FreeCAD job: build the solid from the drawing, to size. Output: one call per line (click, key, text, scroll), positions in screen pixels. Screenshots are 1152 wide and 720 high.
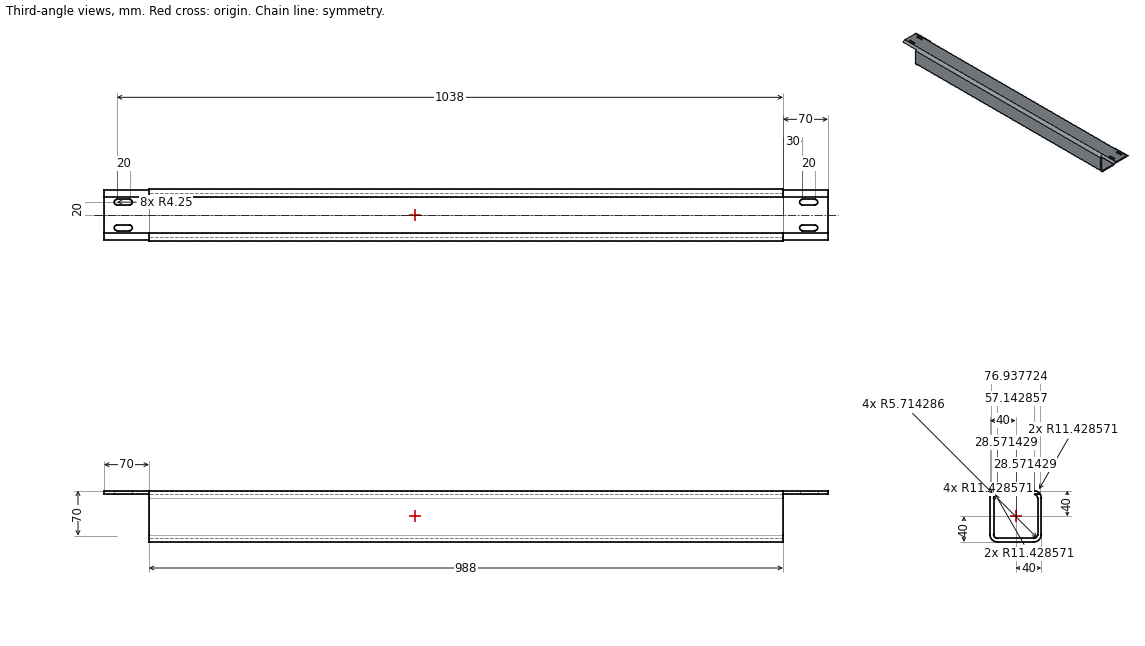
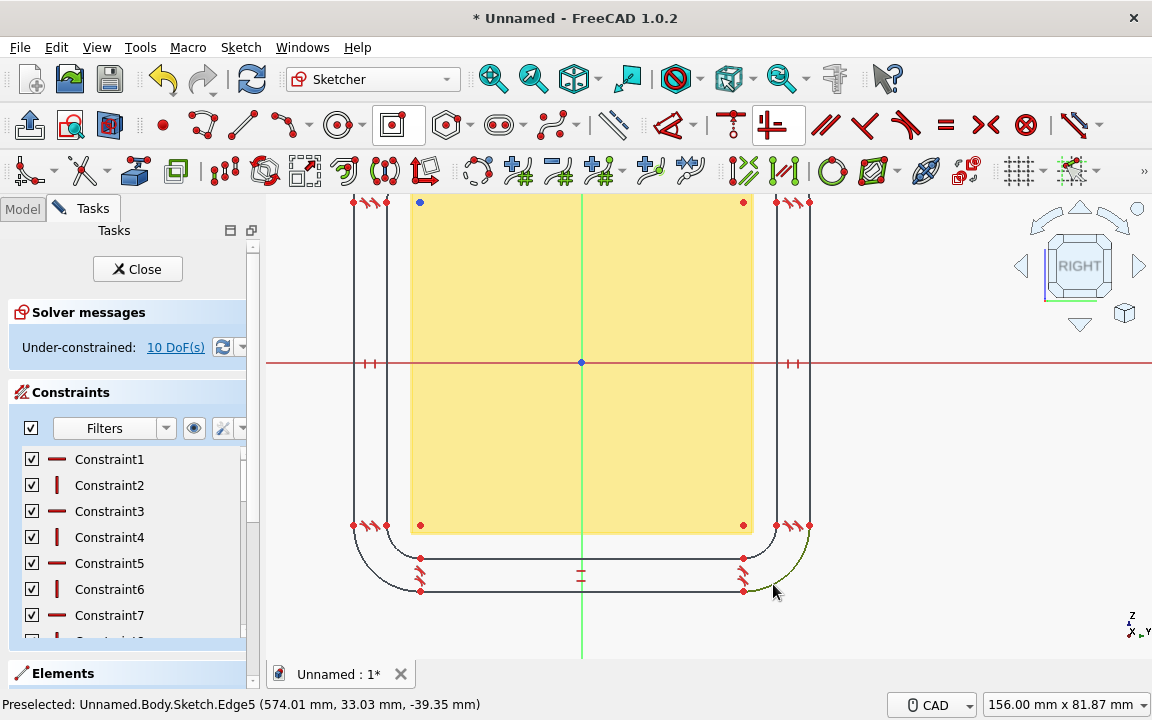
scroll(760, 556, down, 2)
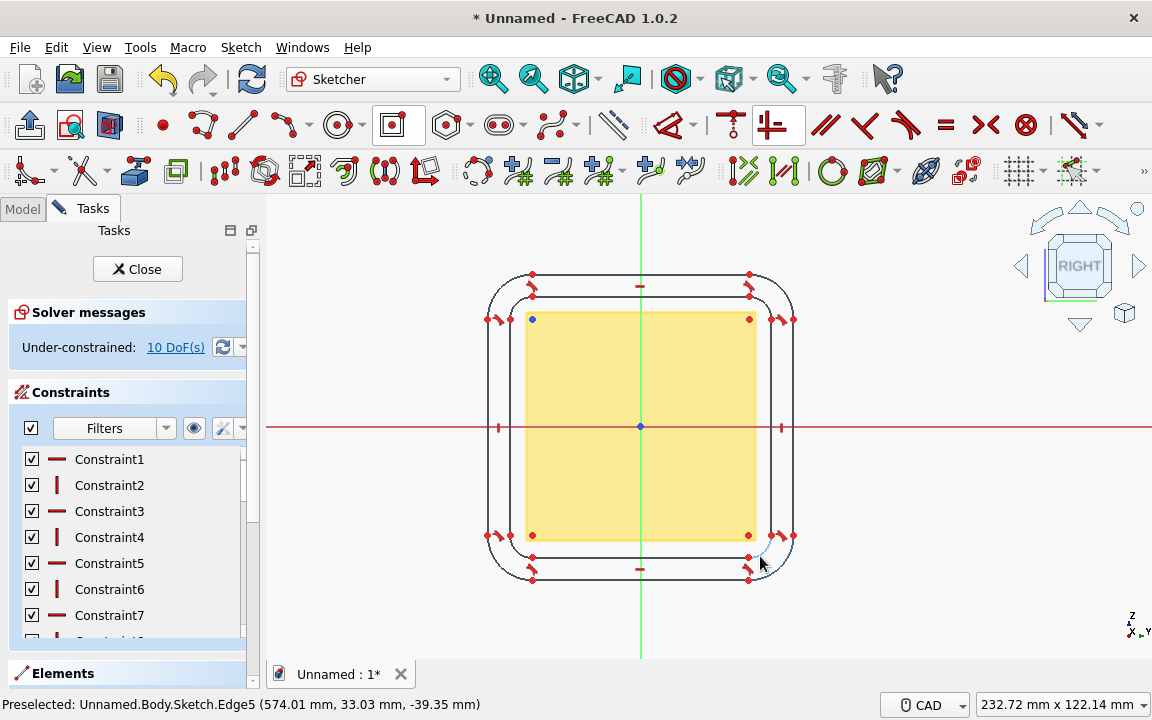
click(789, 299)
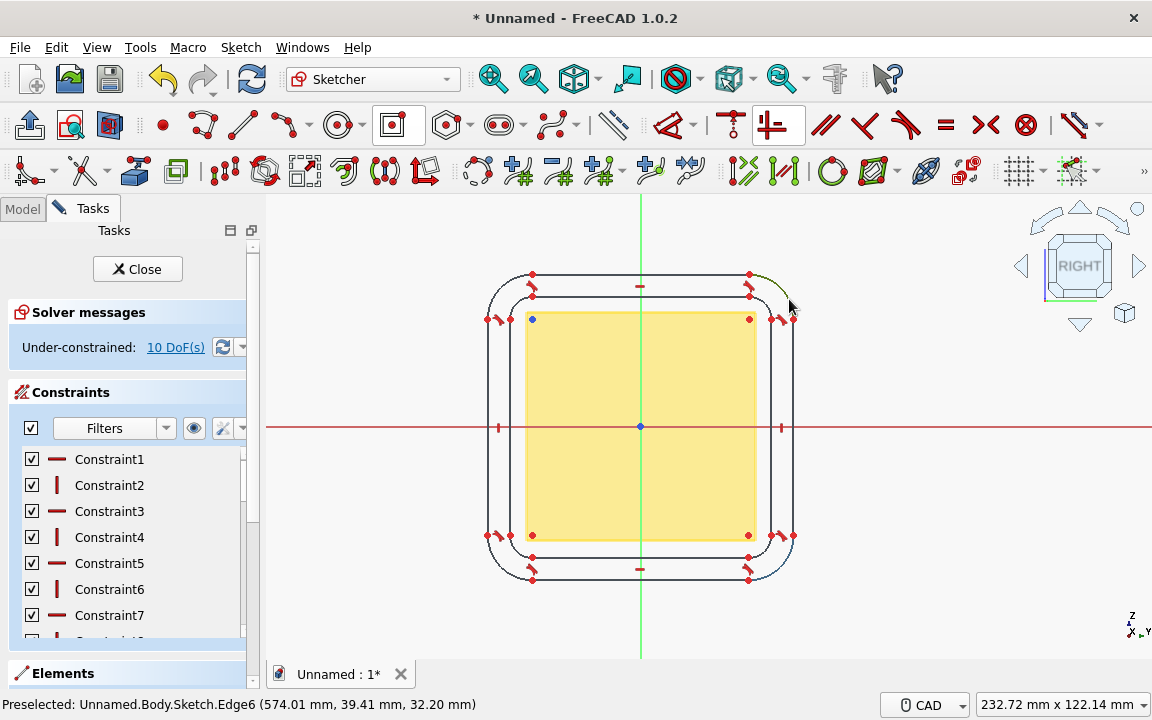
click(512, 280)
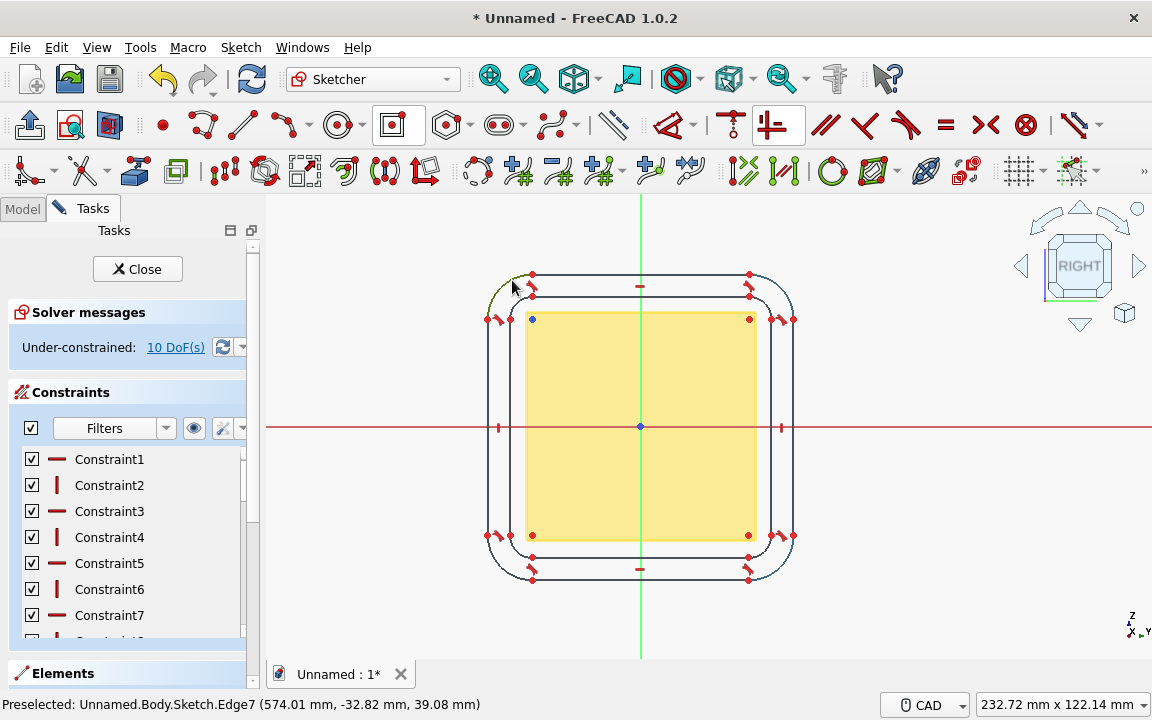
click(493, 556)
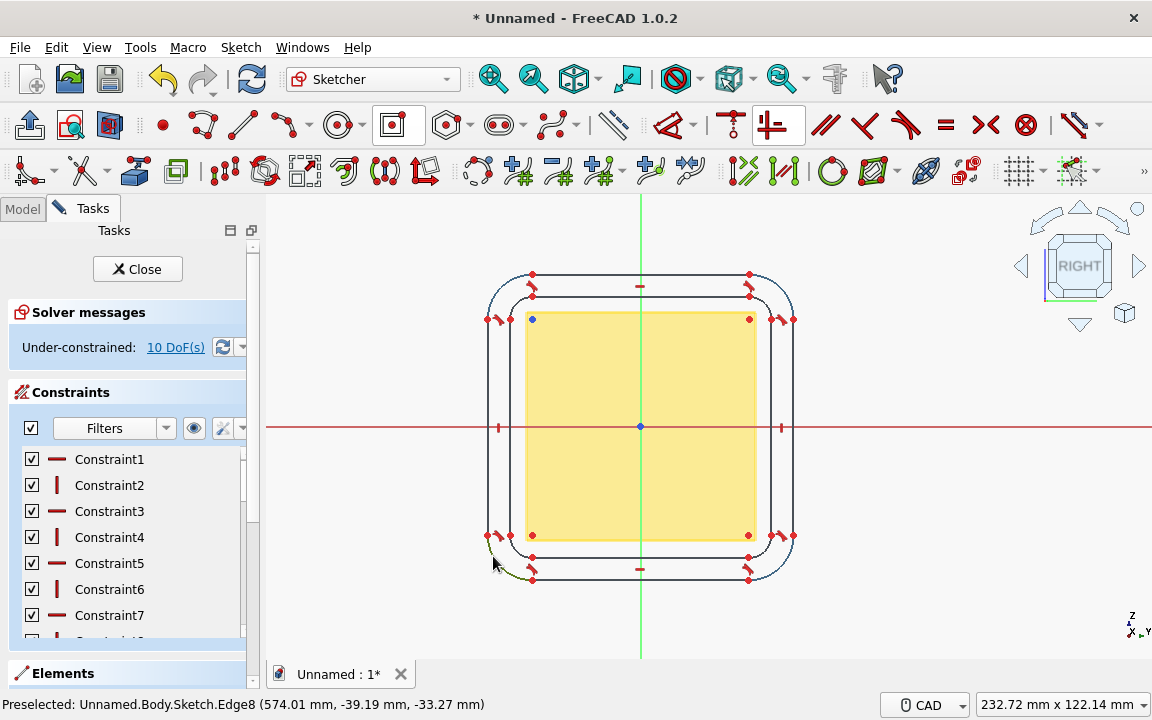
click(946, 126)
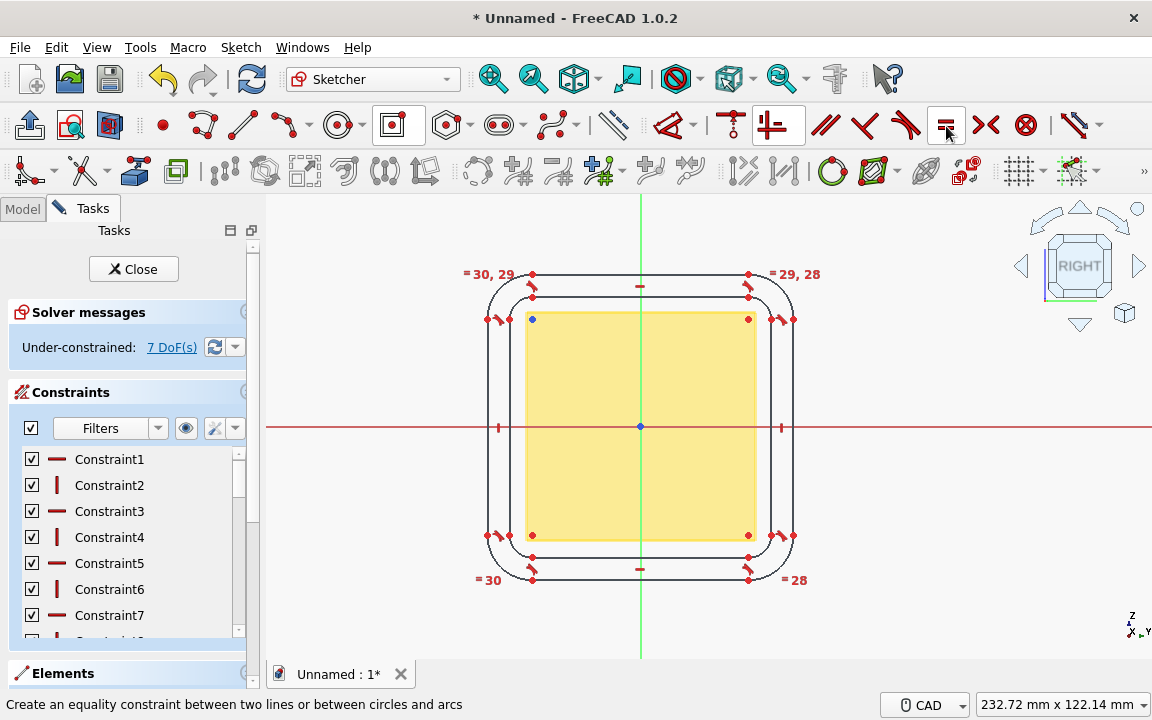
scroll(769, 309, up, 2)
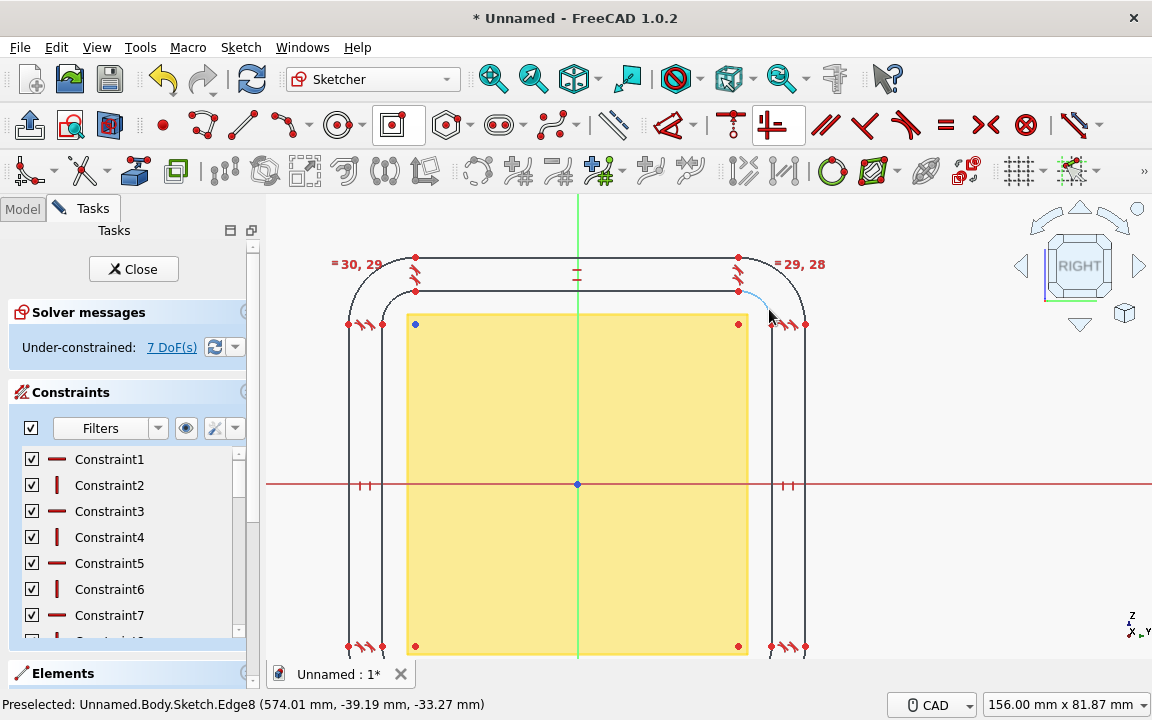
click(768, 309)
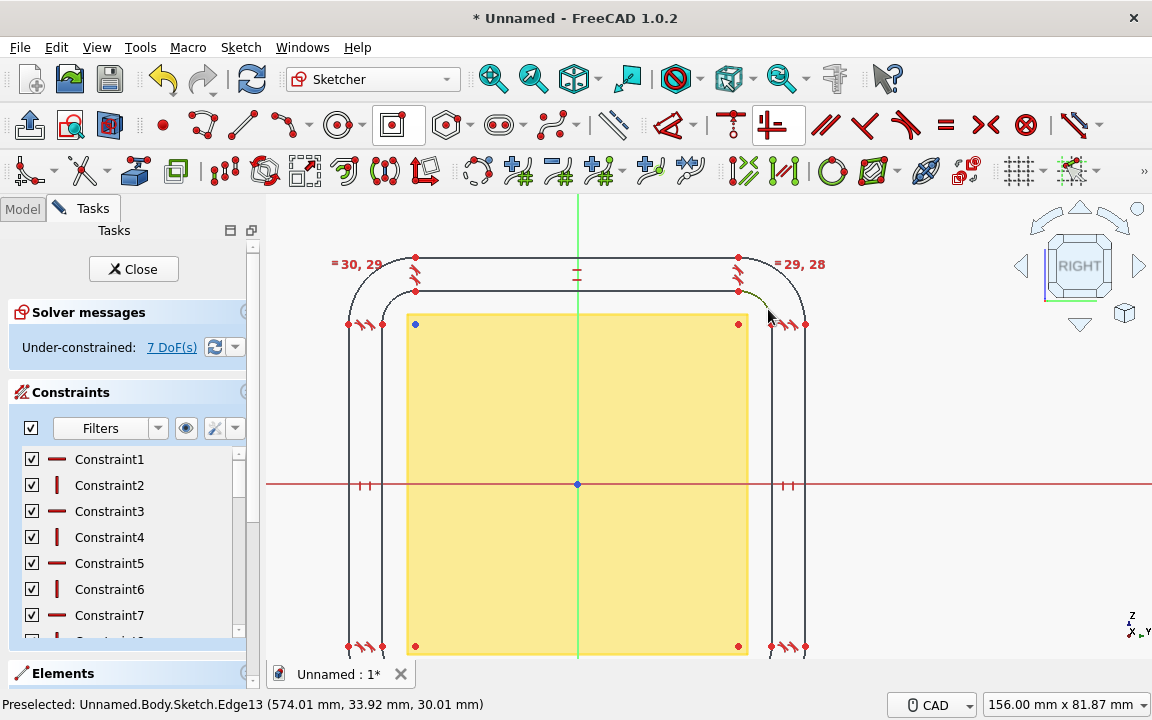
click(400, 295)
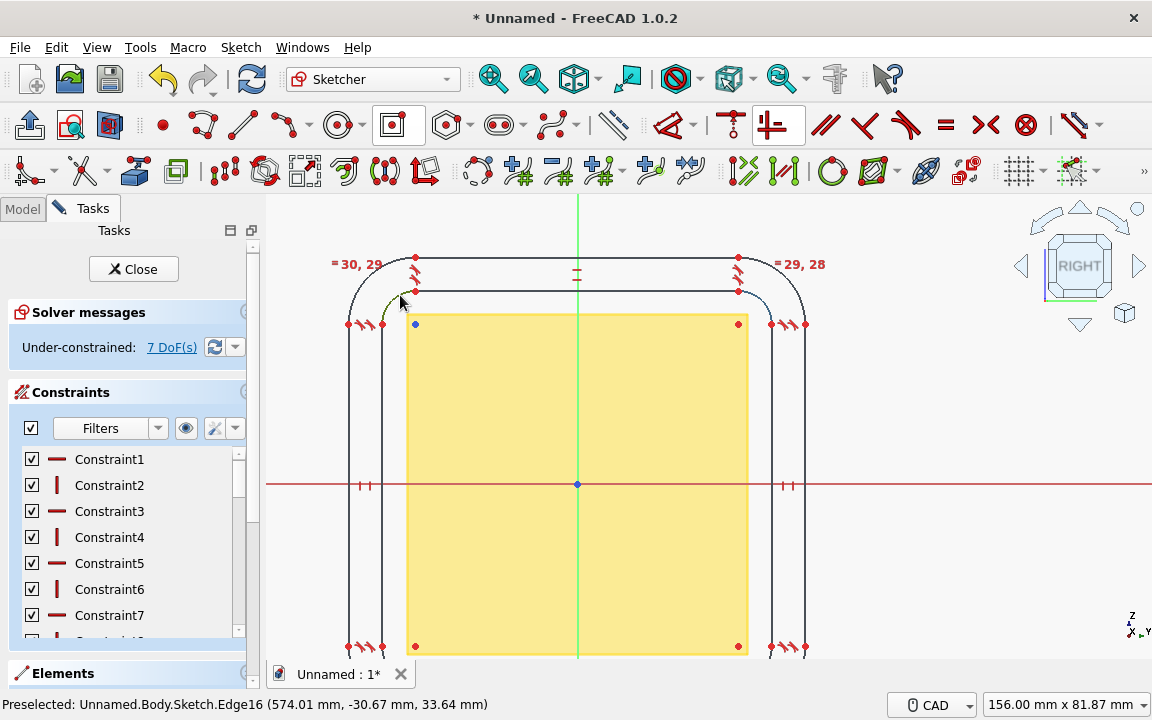
key(e)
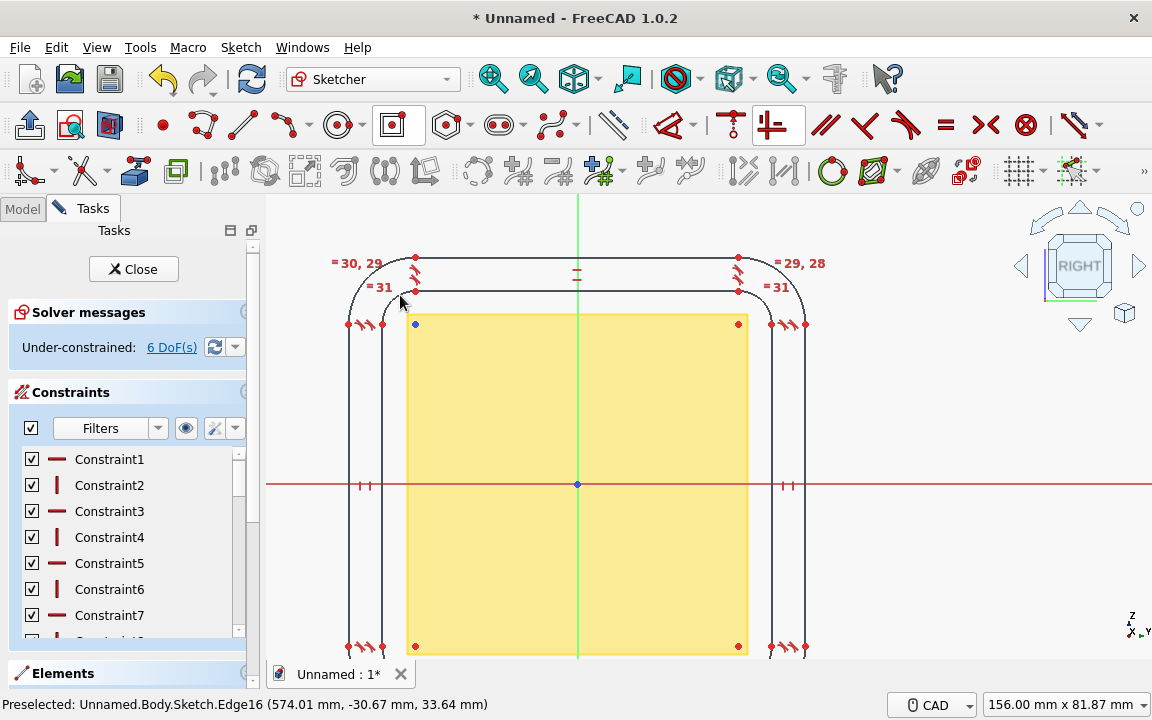
click(668, 126)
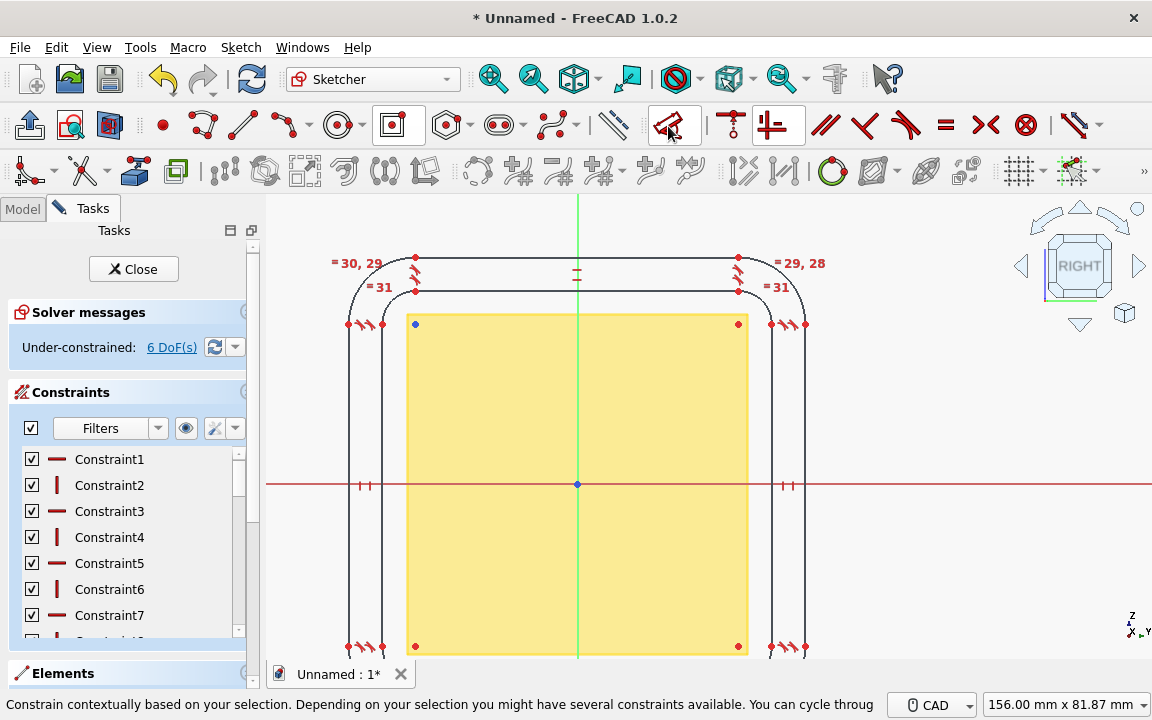
scroll(769, 309, down, 2)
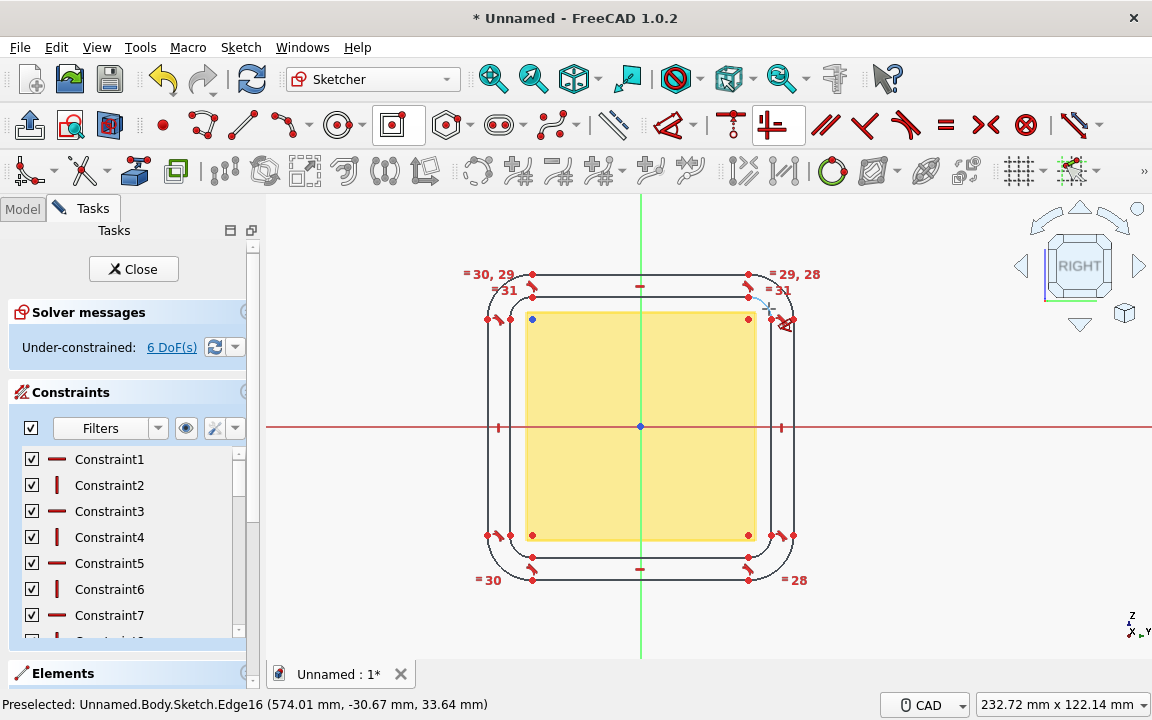
click(769, 575)
click(784, 603)